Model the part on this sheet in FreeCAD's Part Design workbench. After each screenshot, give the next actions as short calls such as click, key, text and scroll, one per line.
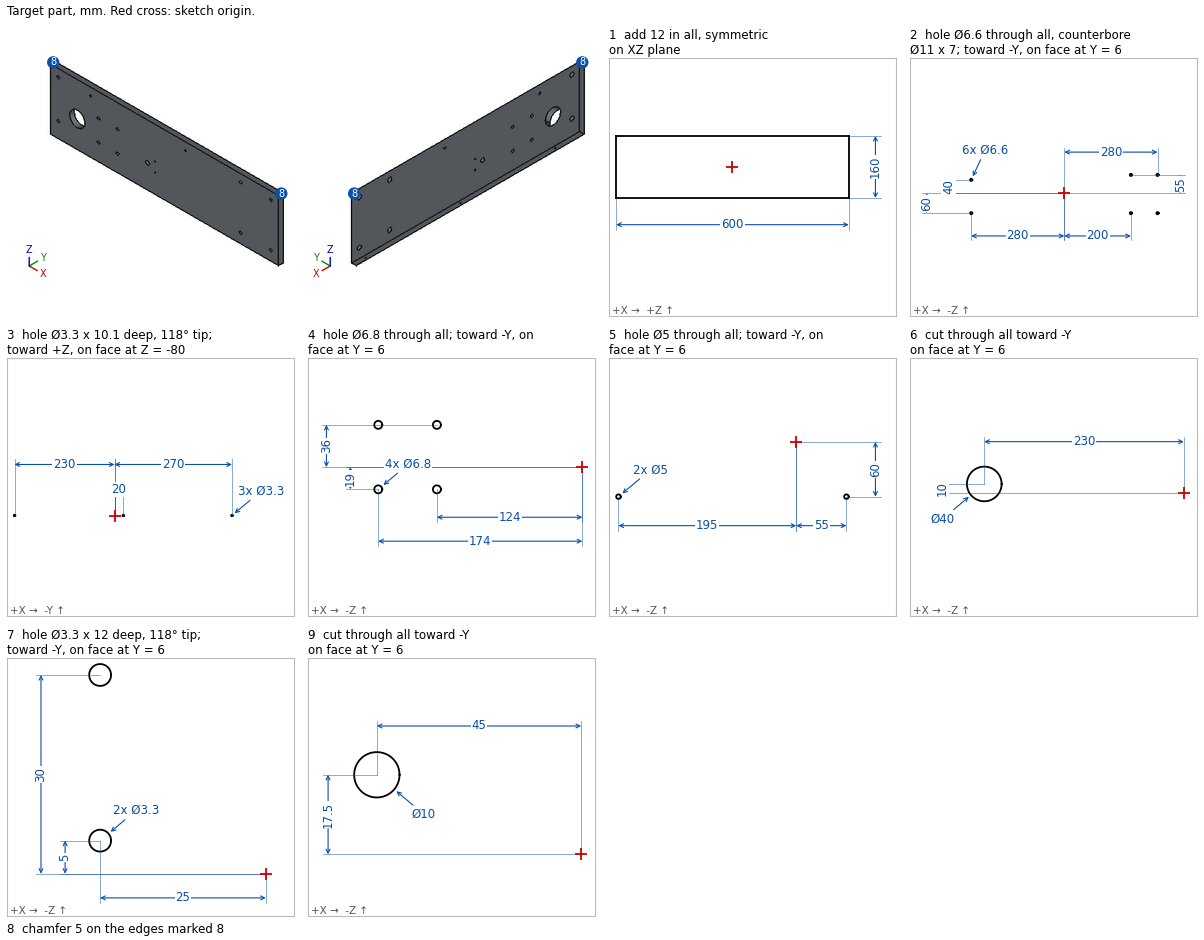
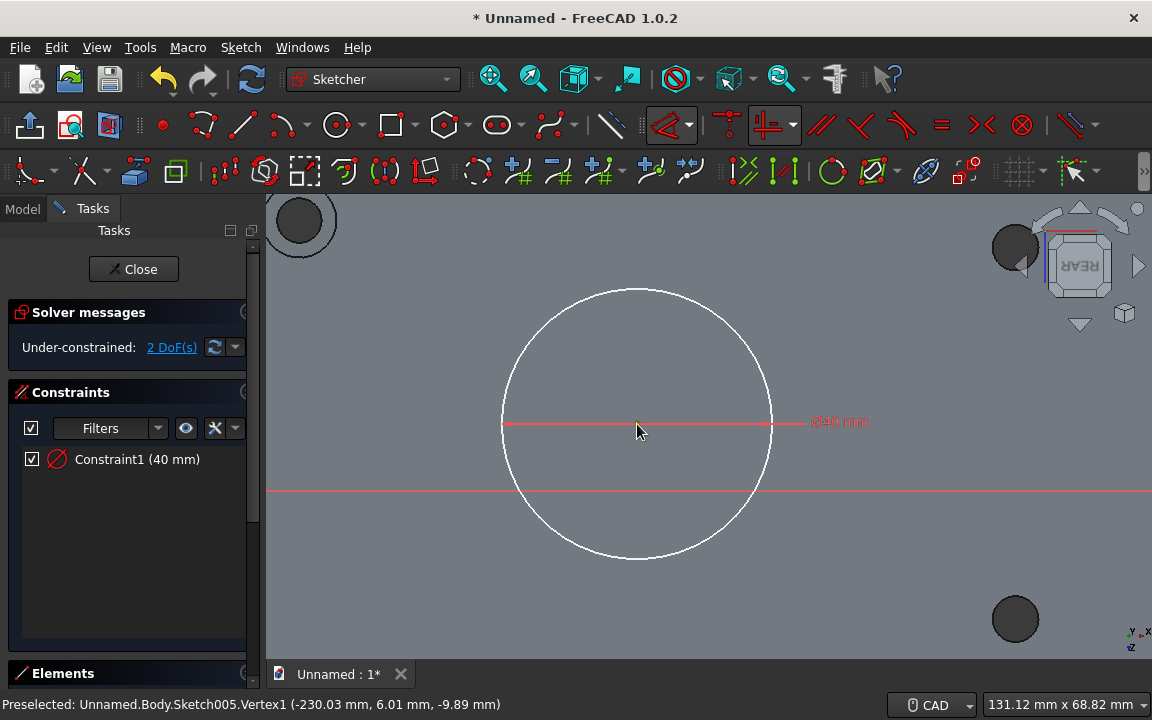
click(692, 126)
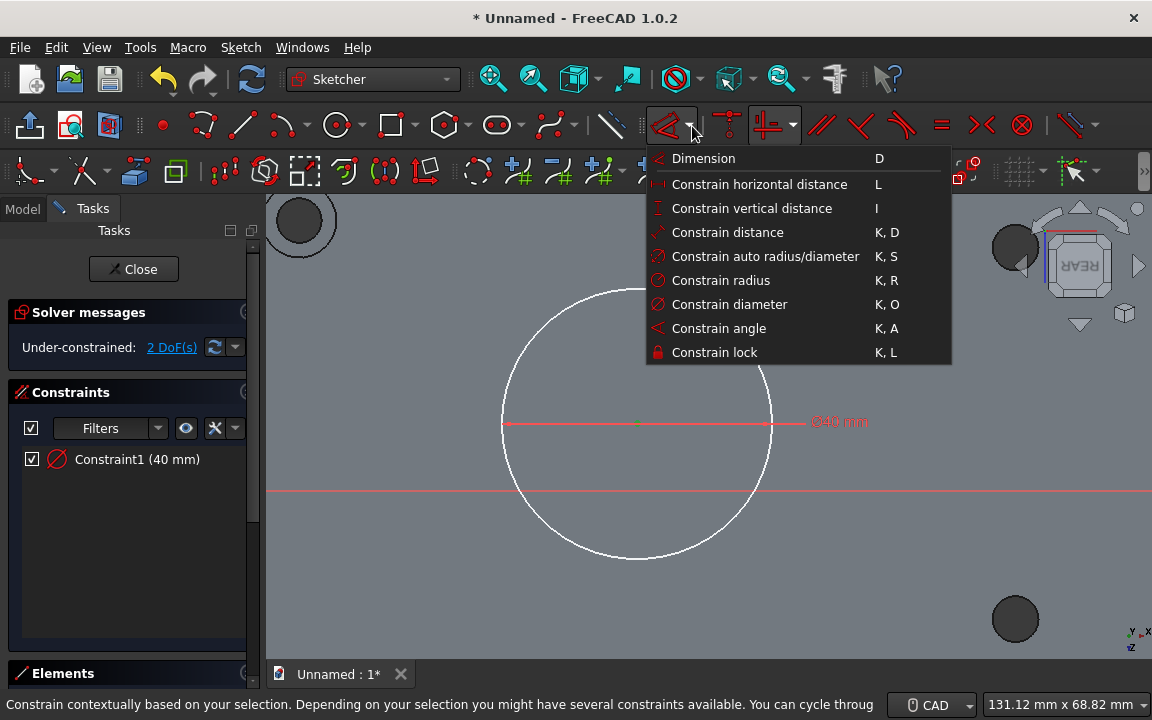
click(799, 208)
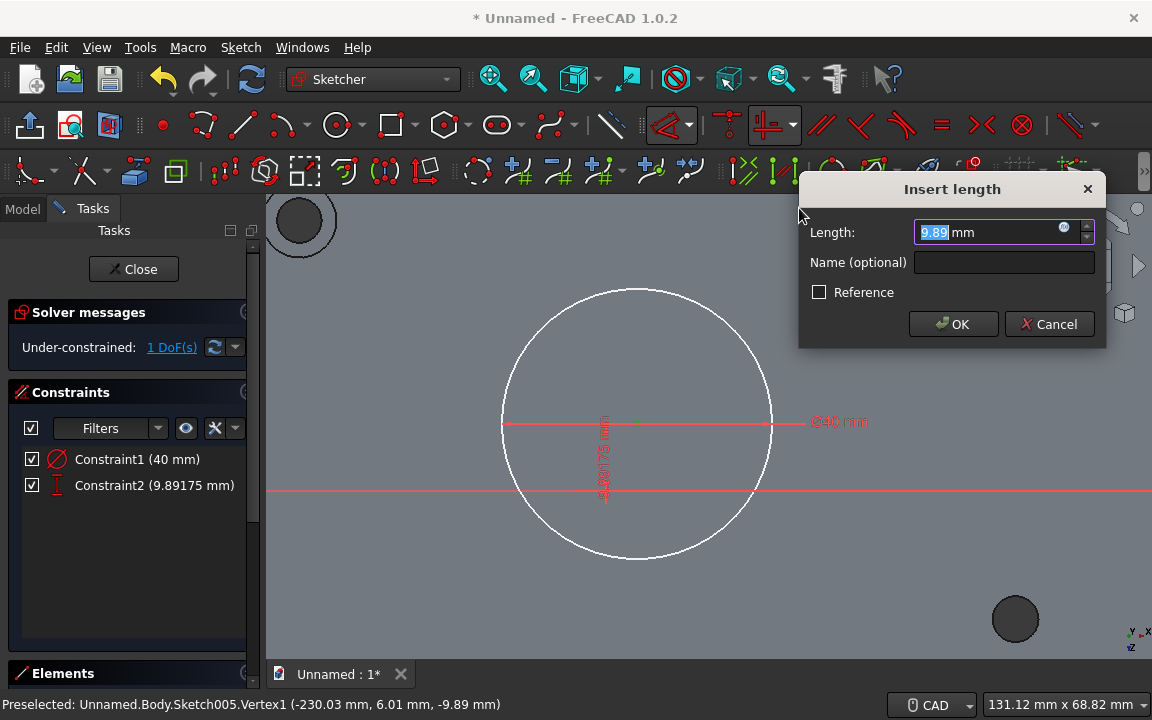
text(10)
key(Return)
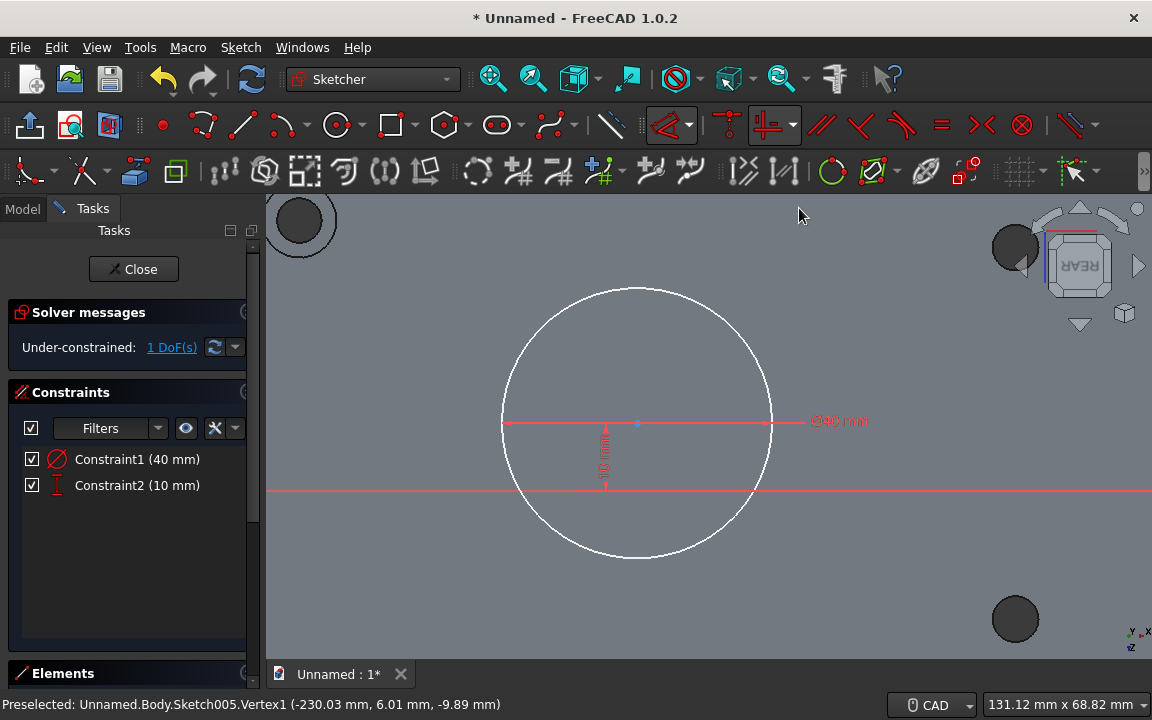
click(637, 423)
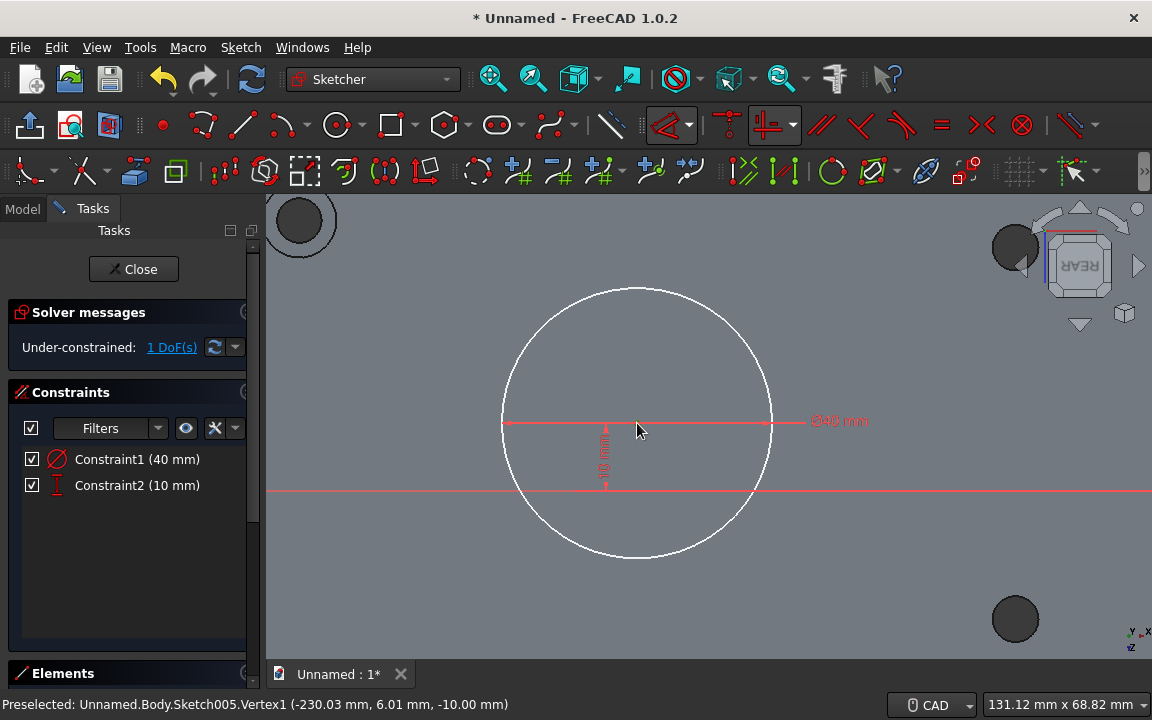
click(692, 126)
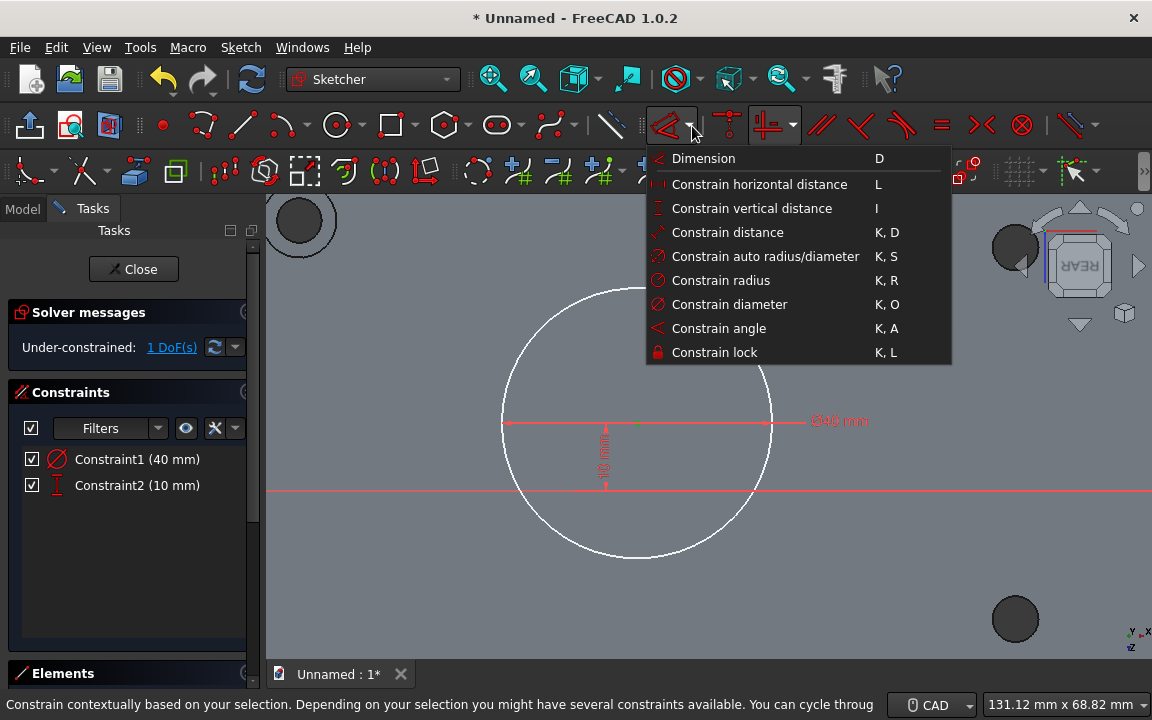
click(799, 184)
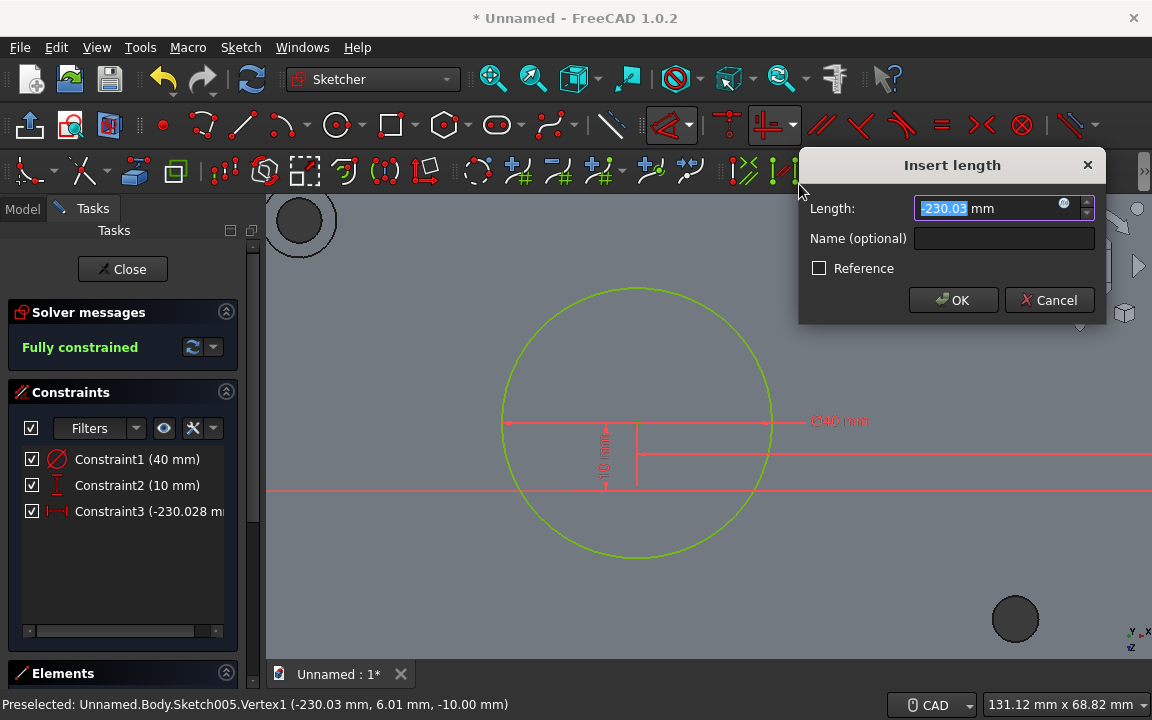
text(-230)
key(Return)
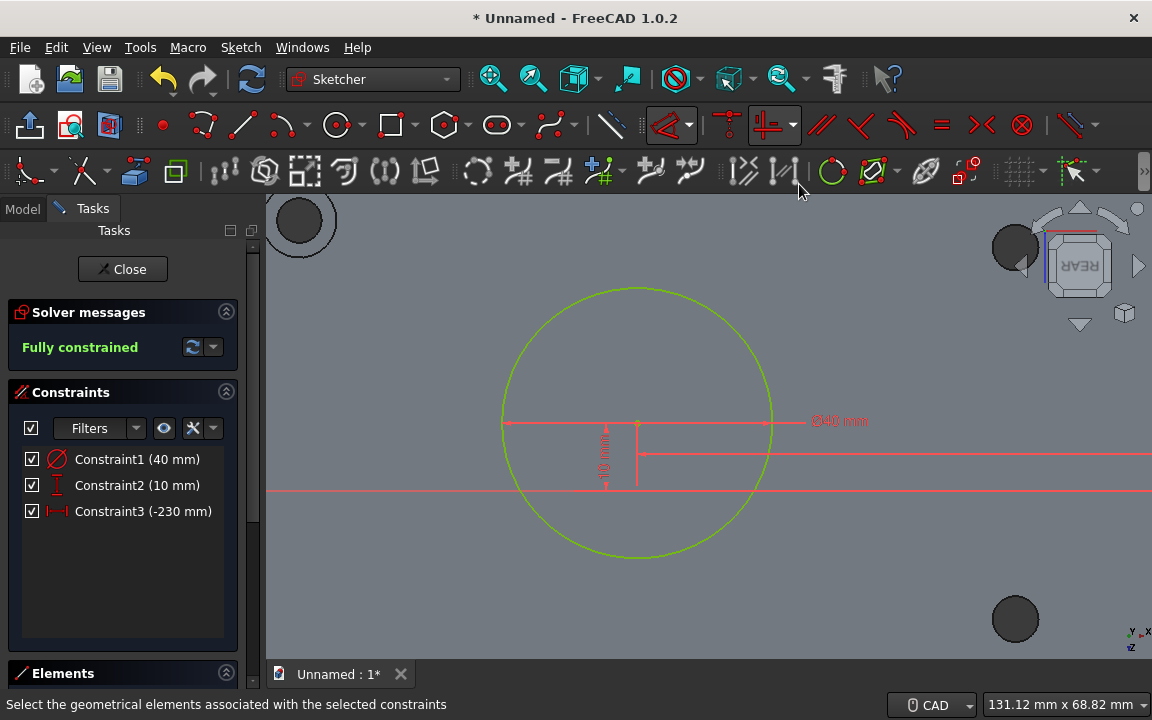
click(123, 269)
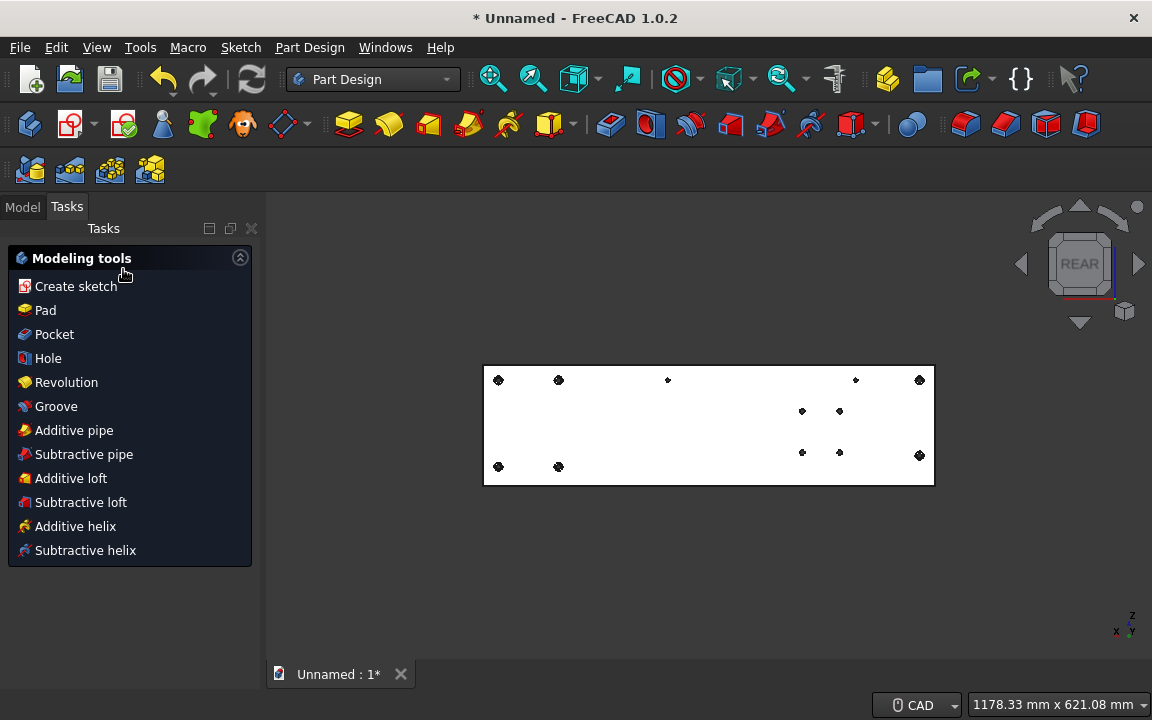
click(612, 124)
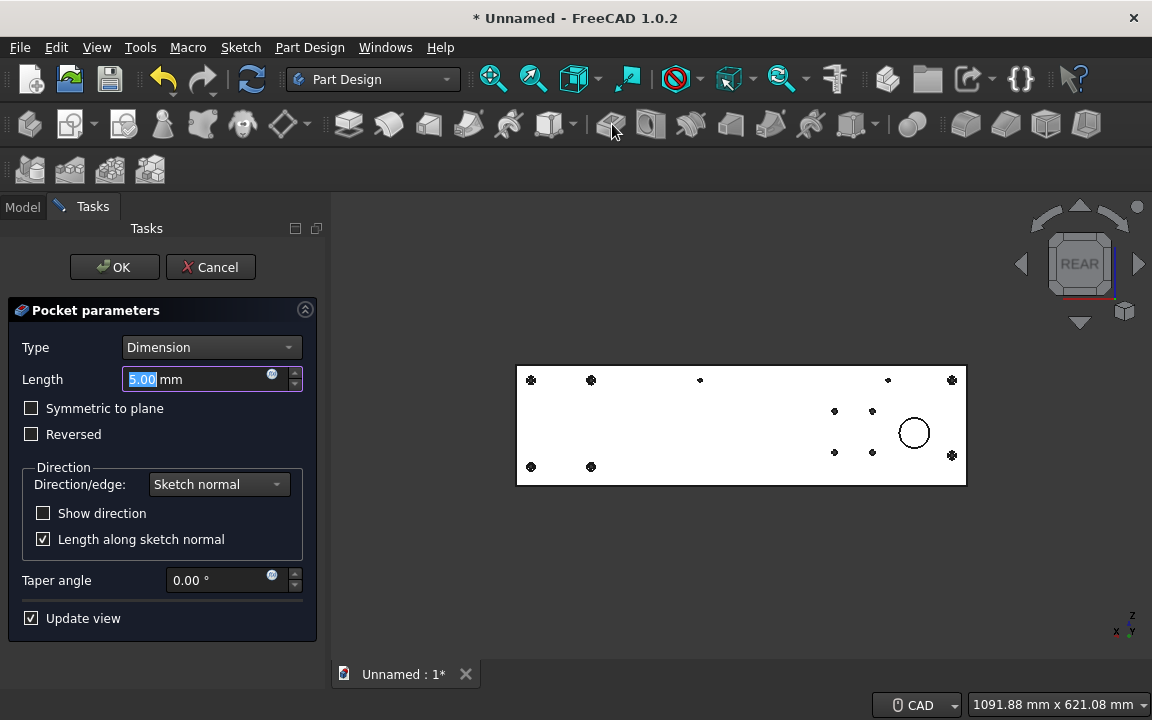
click(212, 348)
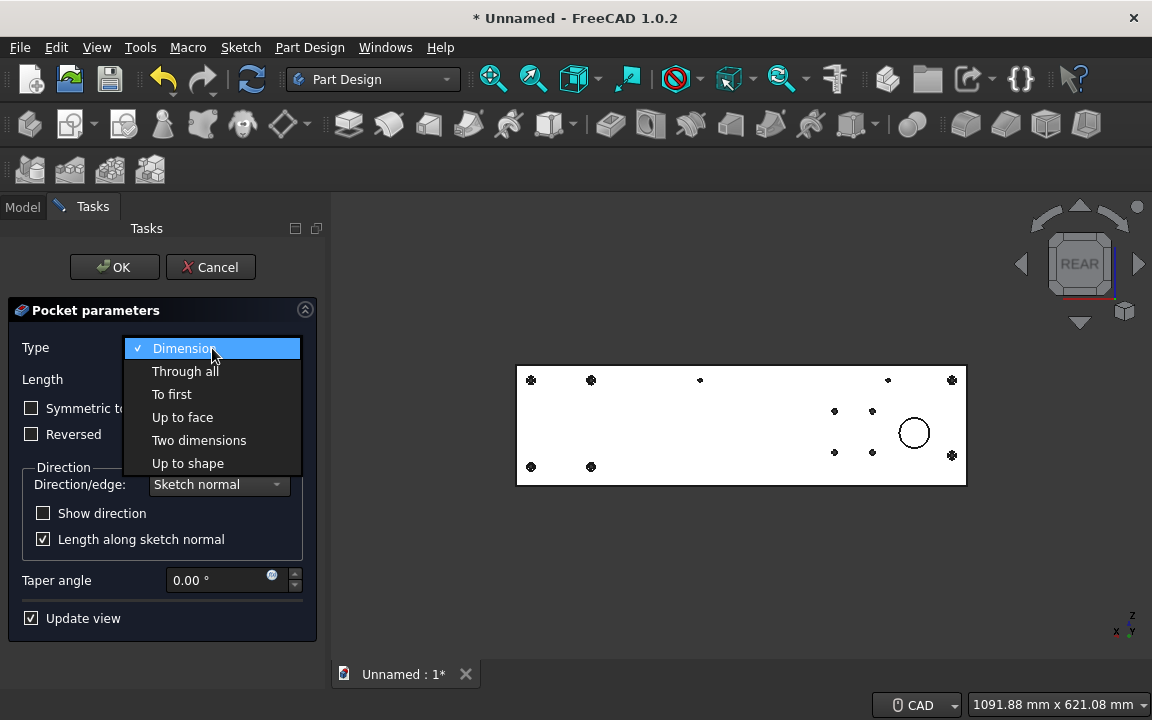
click(212, 372)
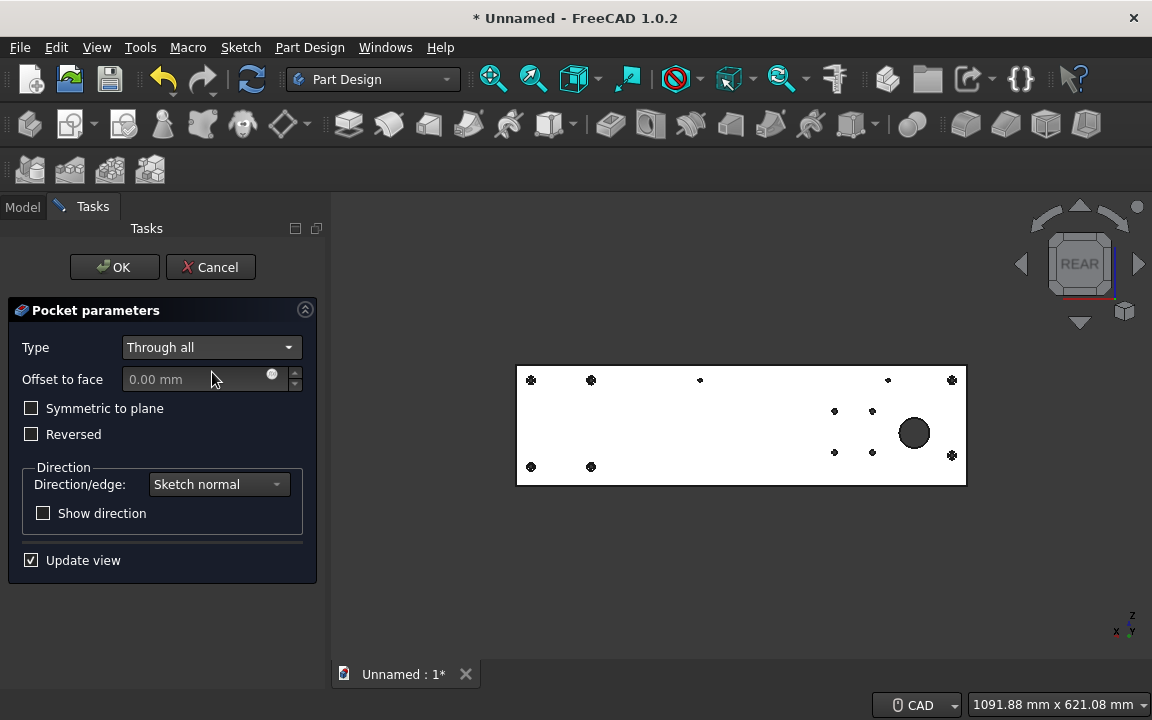
click(115, 267)